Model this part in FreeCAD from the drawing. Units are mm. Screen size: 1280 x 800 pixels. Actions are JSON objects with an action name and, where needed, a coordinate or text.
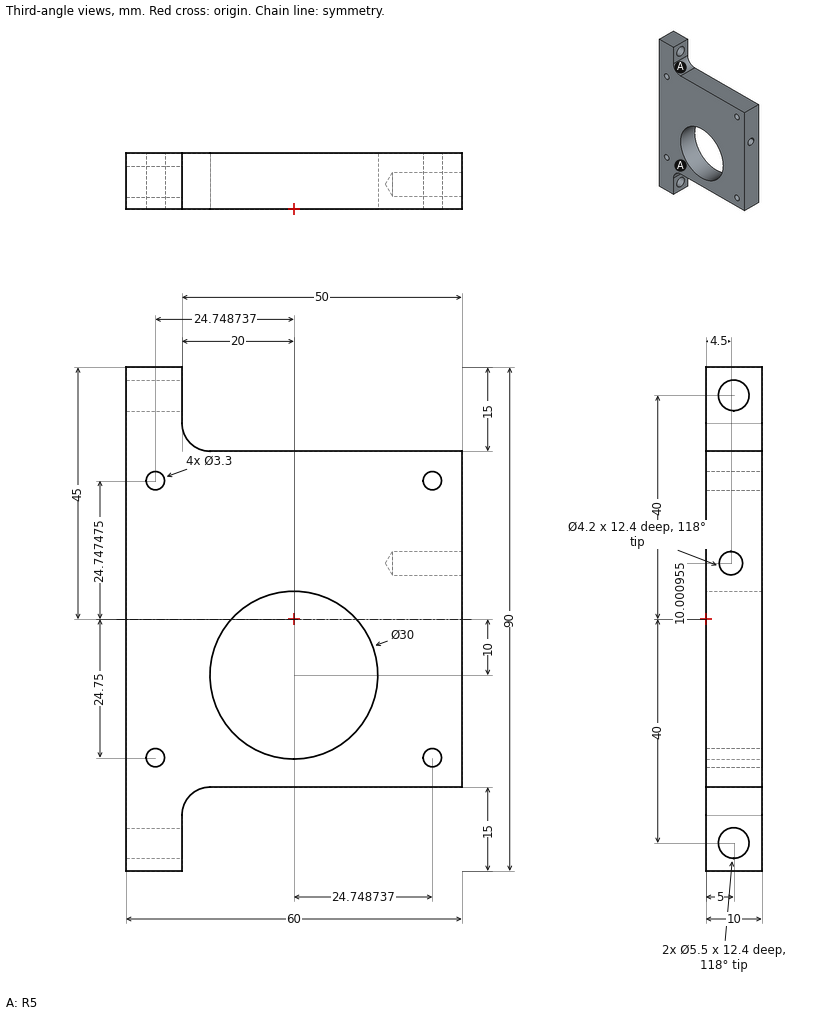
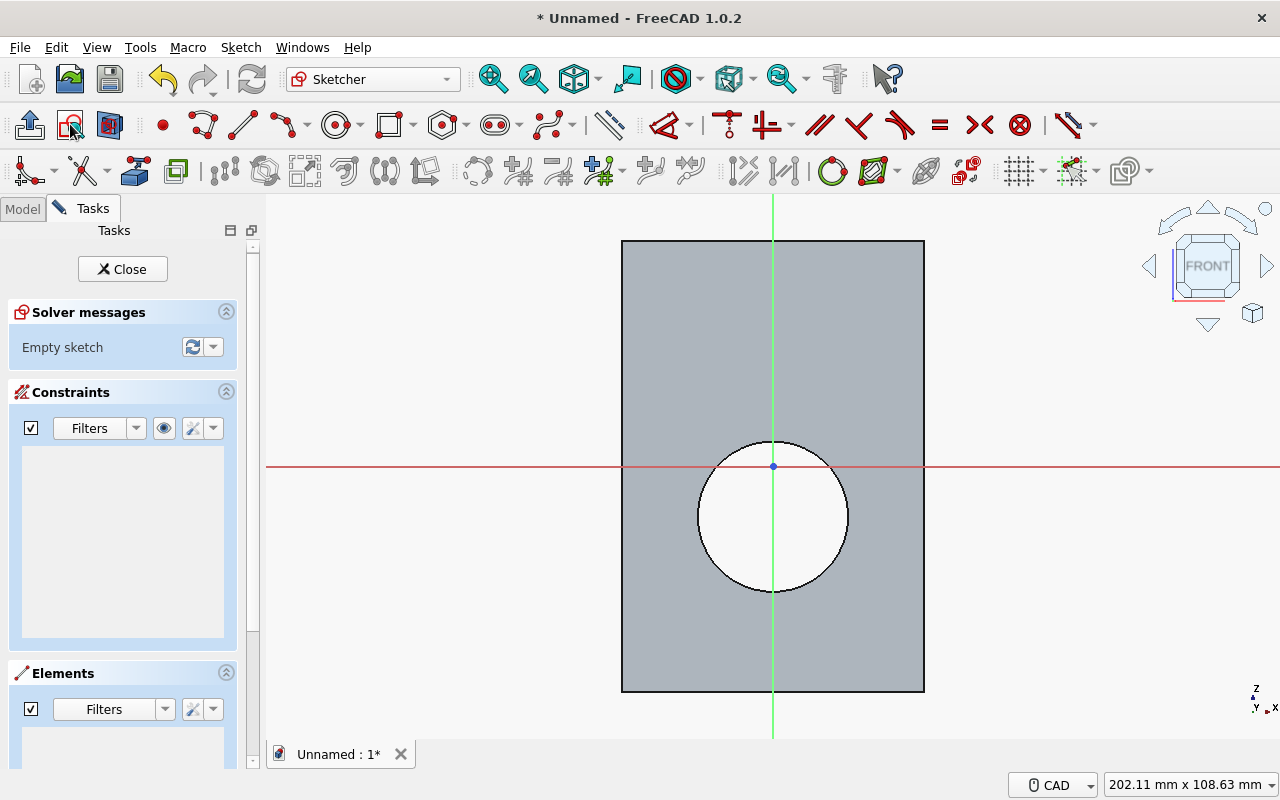
{"action": "key", "text": "g c"}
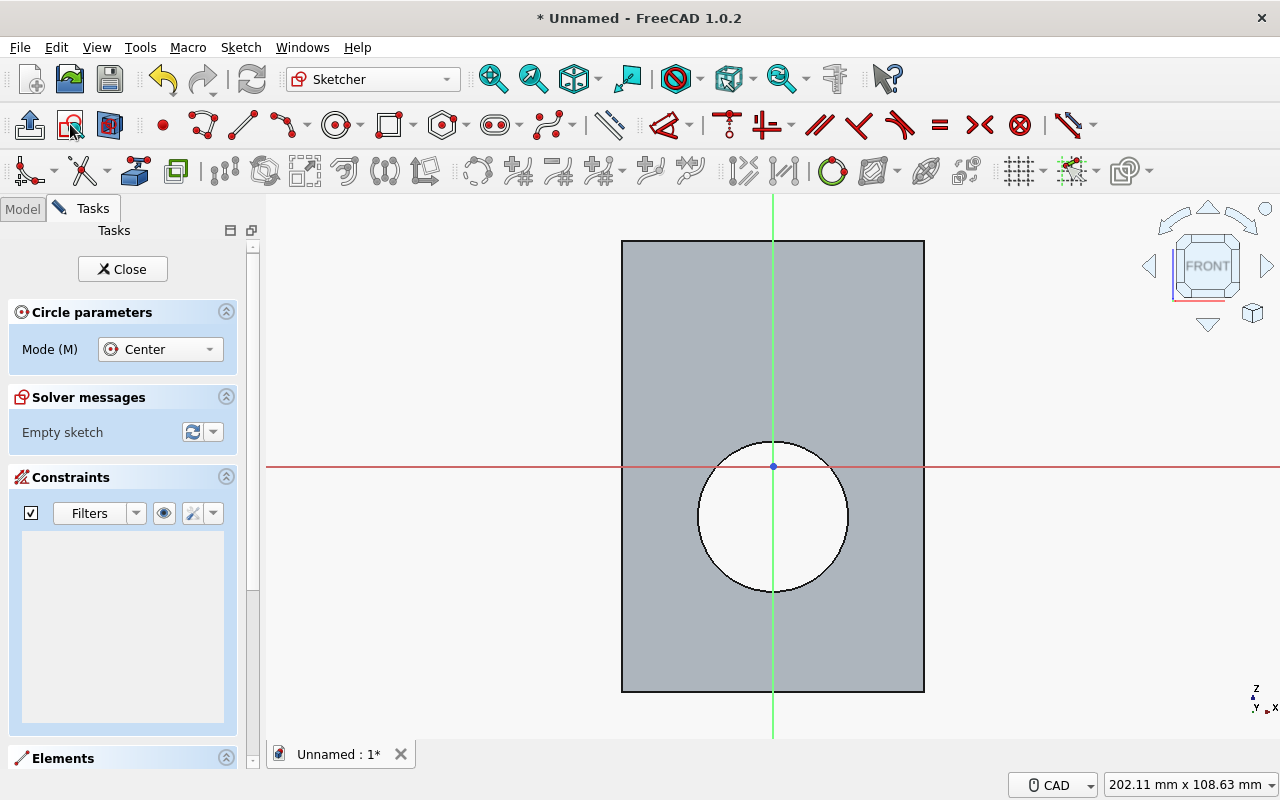
{"action": "scroll", "coordinate": [649, 342], "scroll_direction": "up", "scroll_amount": 6}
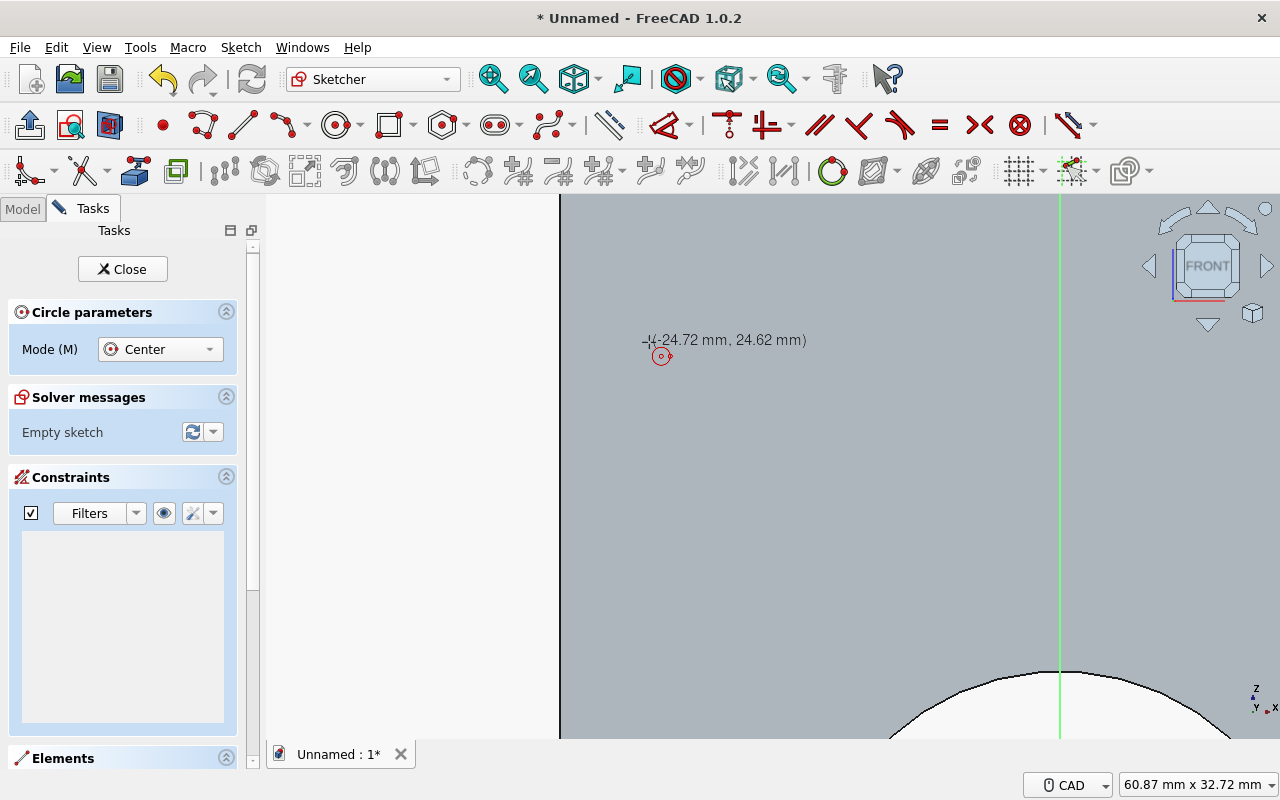
{"action": "left_click", "coordinate": [648, 342]}
{"action": "mouse_move", "coordinate": [667, 323]}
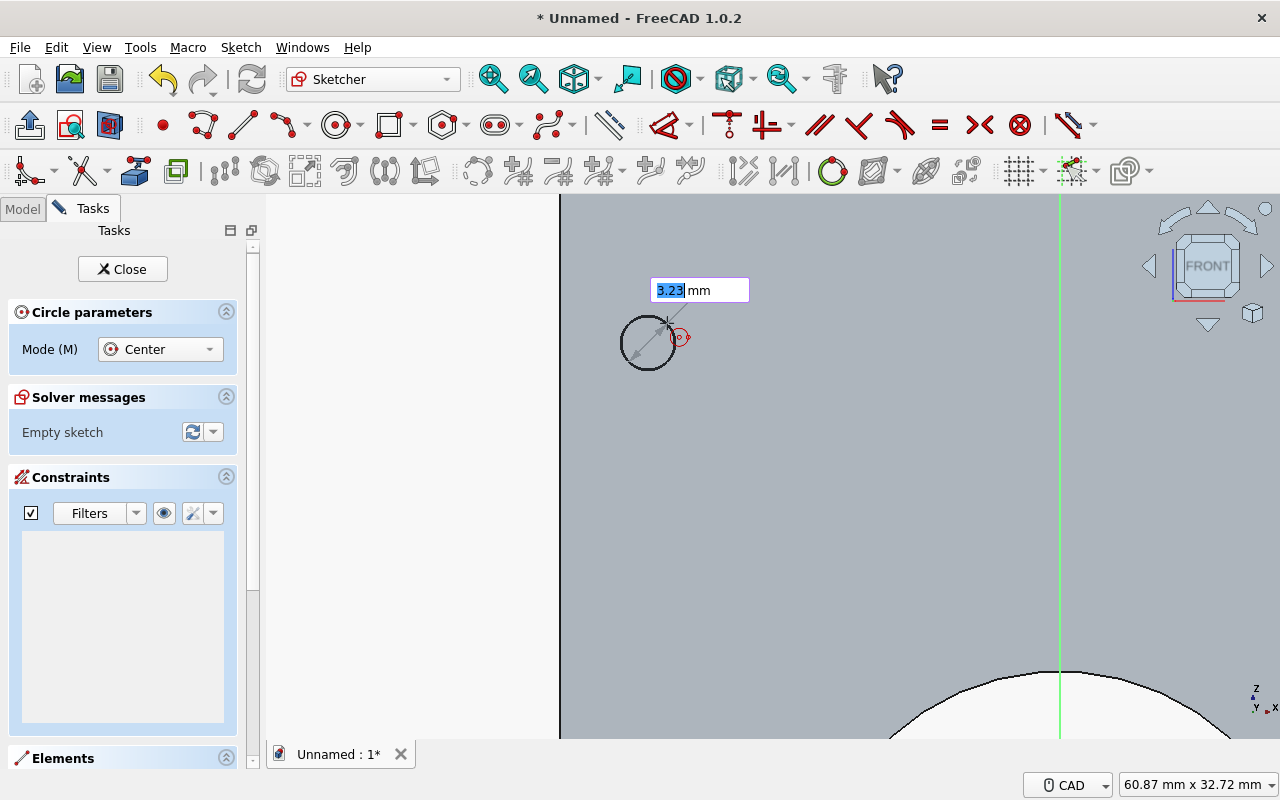
{"action": "type", "text": "3.3"}
{"action": "key", "text": "Return"}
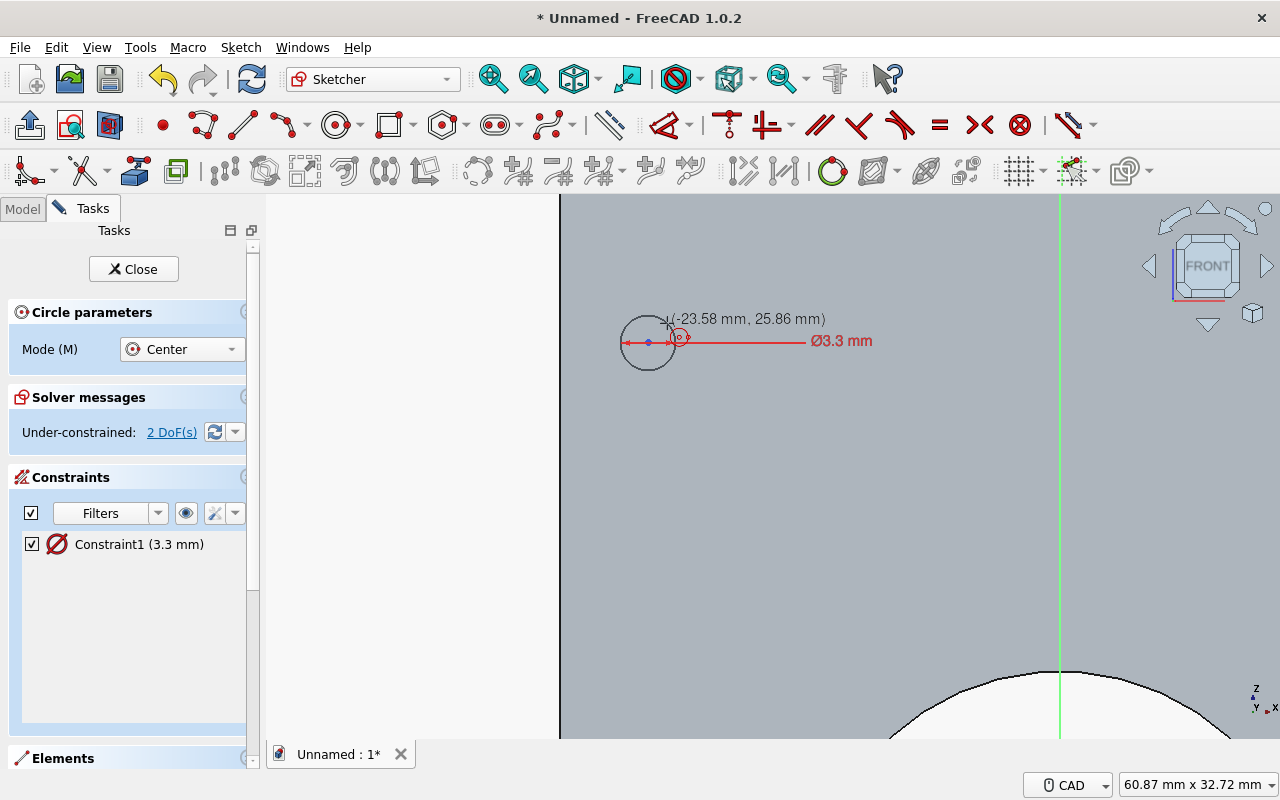
{"action": "scroll", "coordinate": [498, 299], "scroll_direction": "down", "scroll_amount": 5}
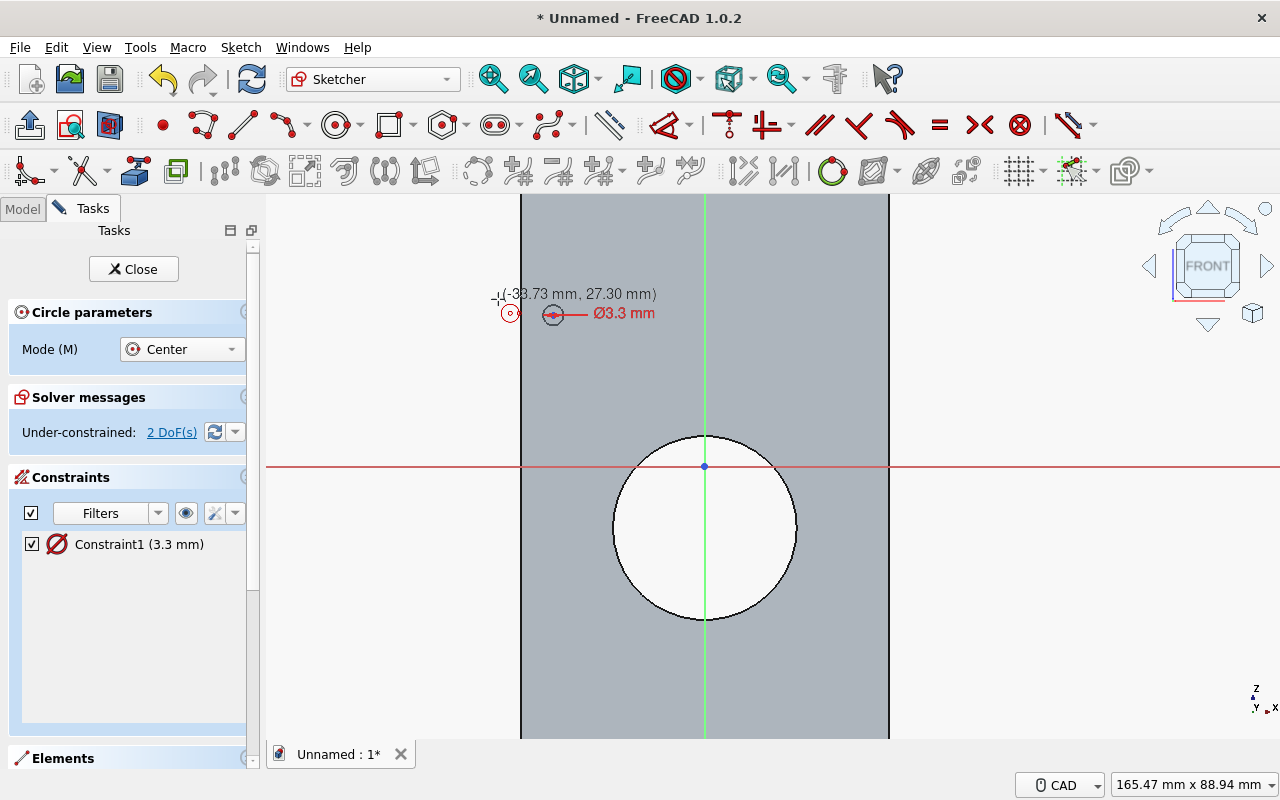
{"action": "scroll", "coordinate": [553, 618], "scroll_direction": "up", "scroll_amount": 5}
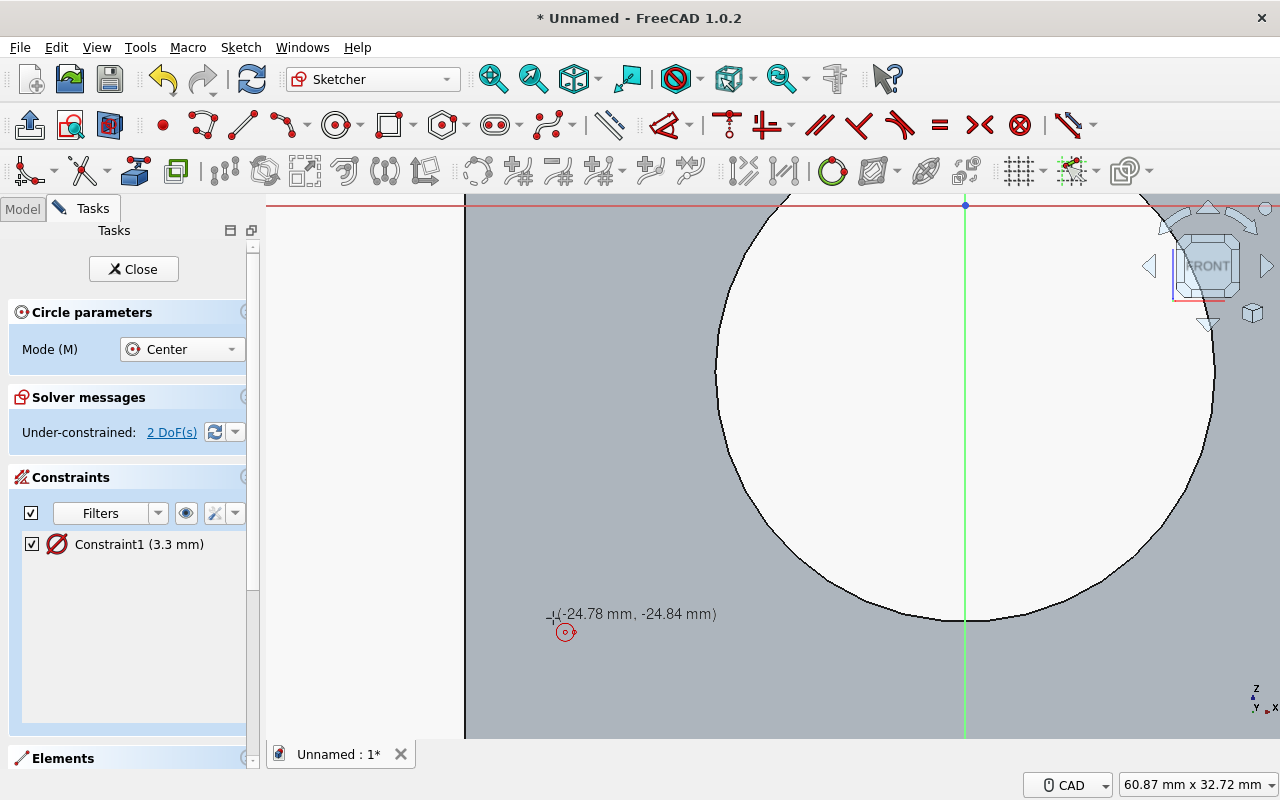
{"action": "left_click", "coordinate": [553, 618]}
{"action": "mouse_move", "coordinate": [572, 598]}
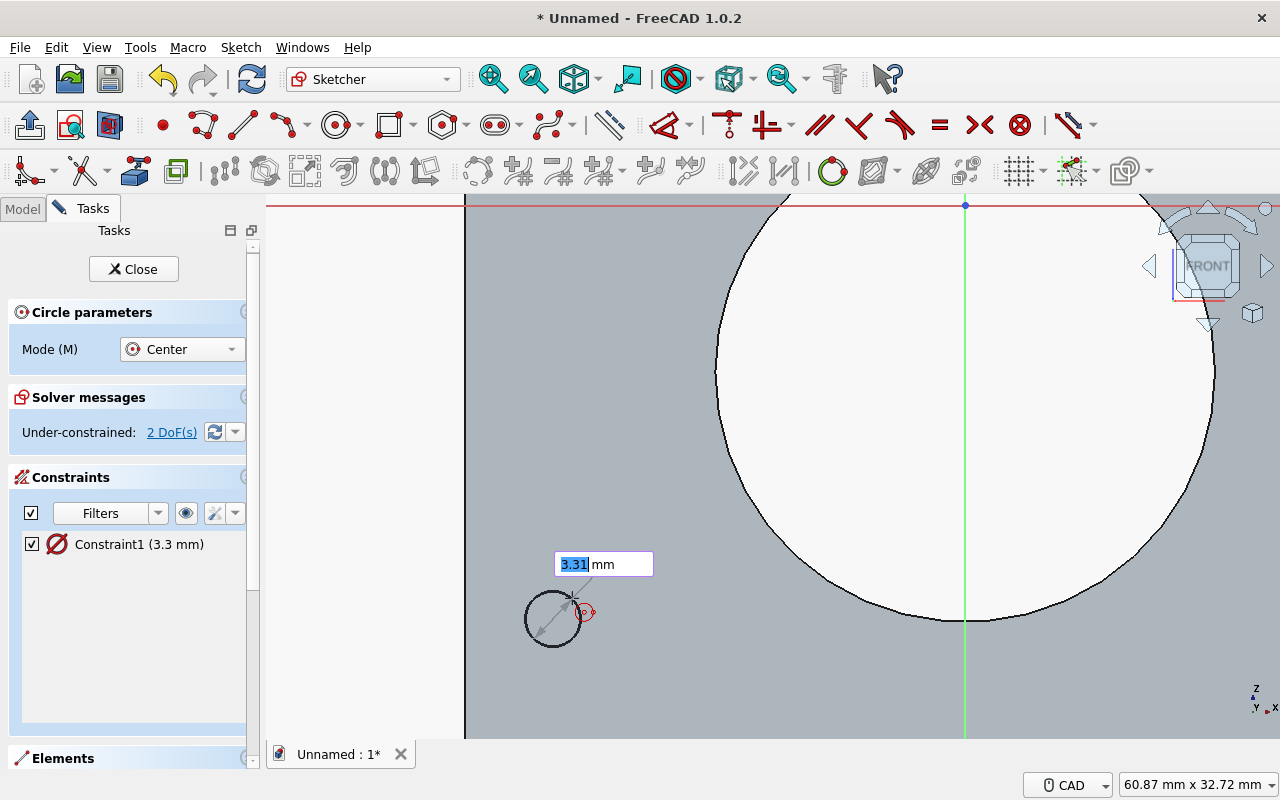
{"action": "type", "text": "3.3"}
{"action": "key", "text": "Return"}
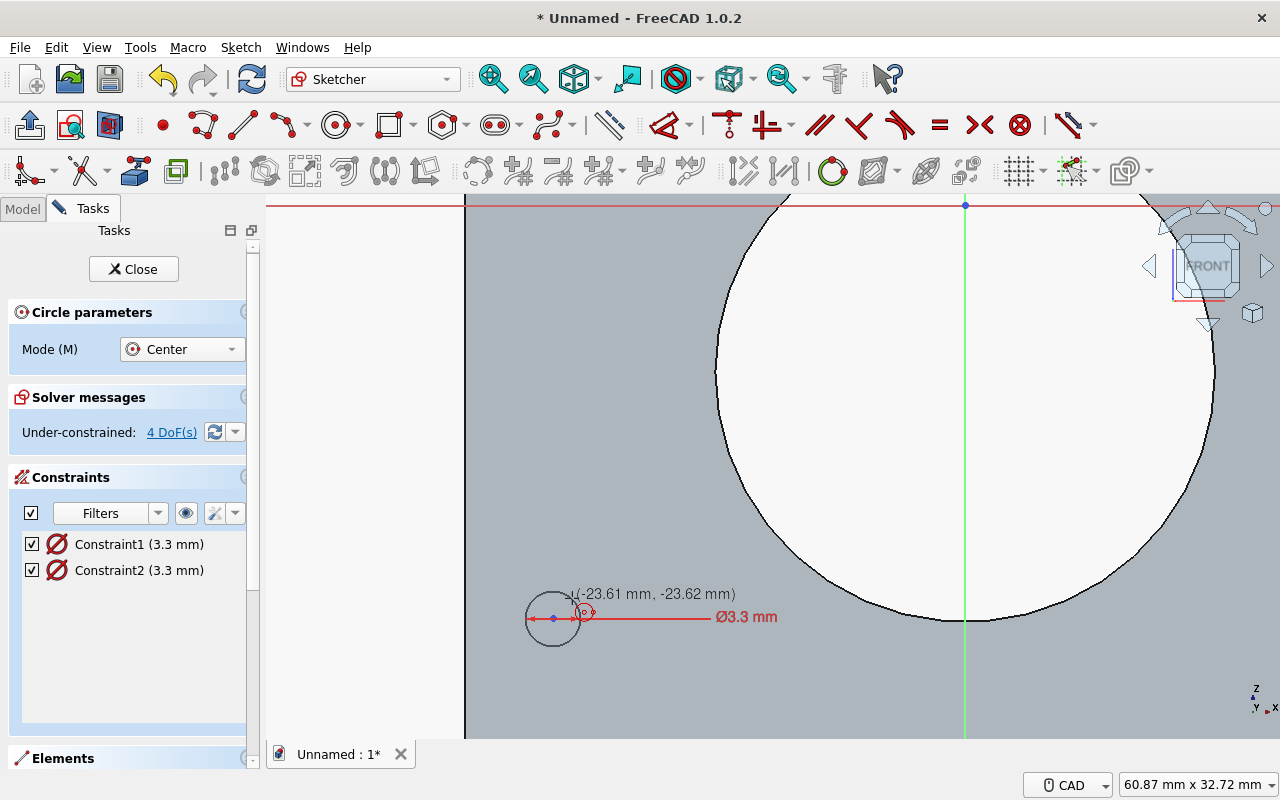
{"action": "scroll", "coordinate": [553, 618], "scroll_direction": "down", "scroll_amount": 5}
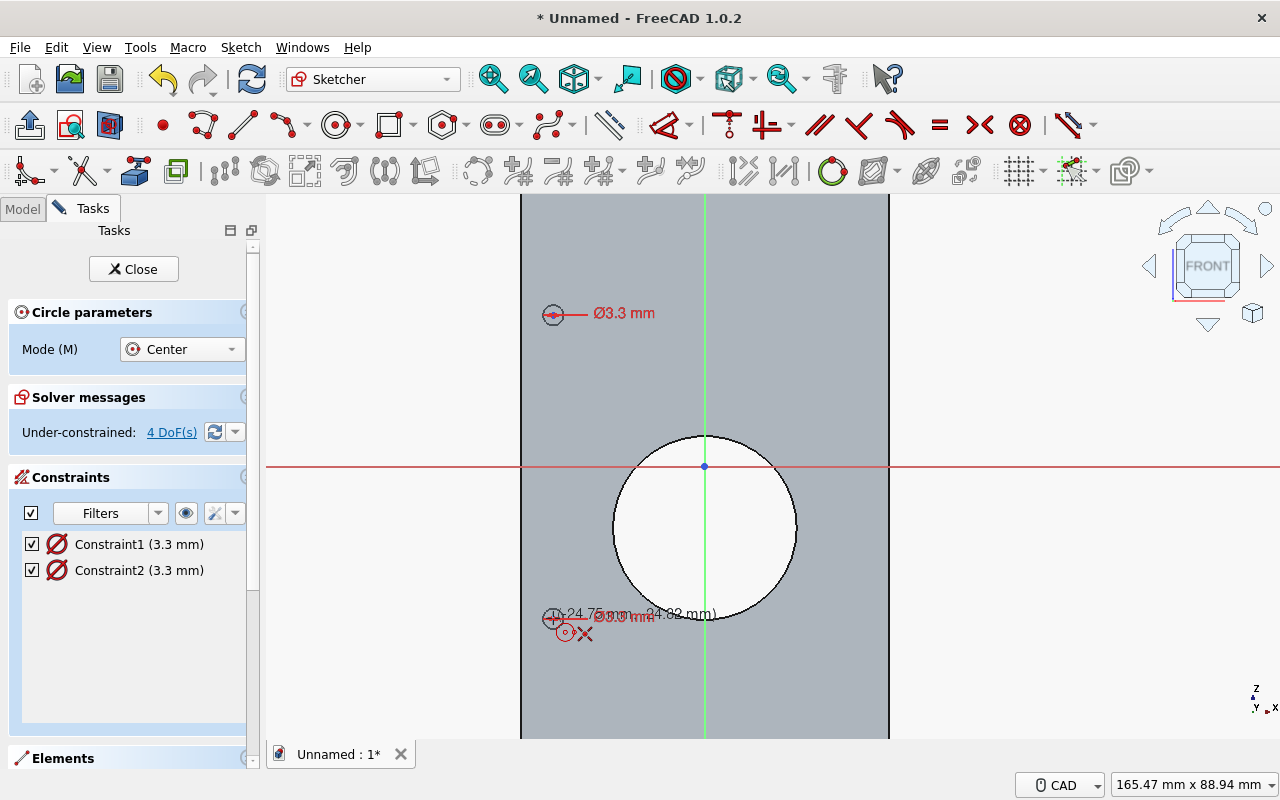
{"action": "scroll", "coordinate": [856, 618], "scroll_direction": "up", "scroll_amount": 5}